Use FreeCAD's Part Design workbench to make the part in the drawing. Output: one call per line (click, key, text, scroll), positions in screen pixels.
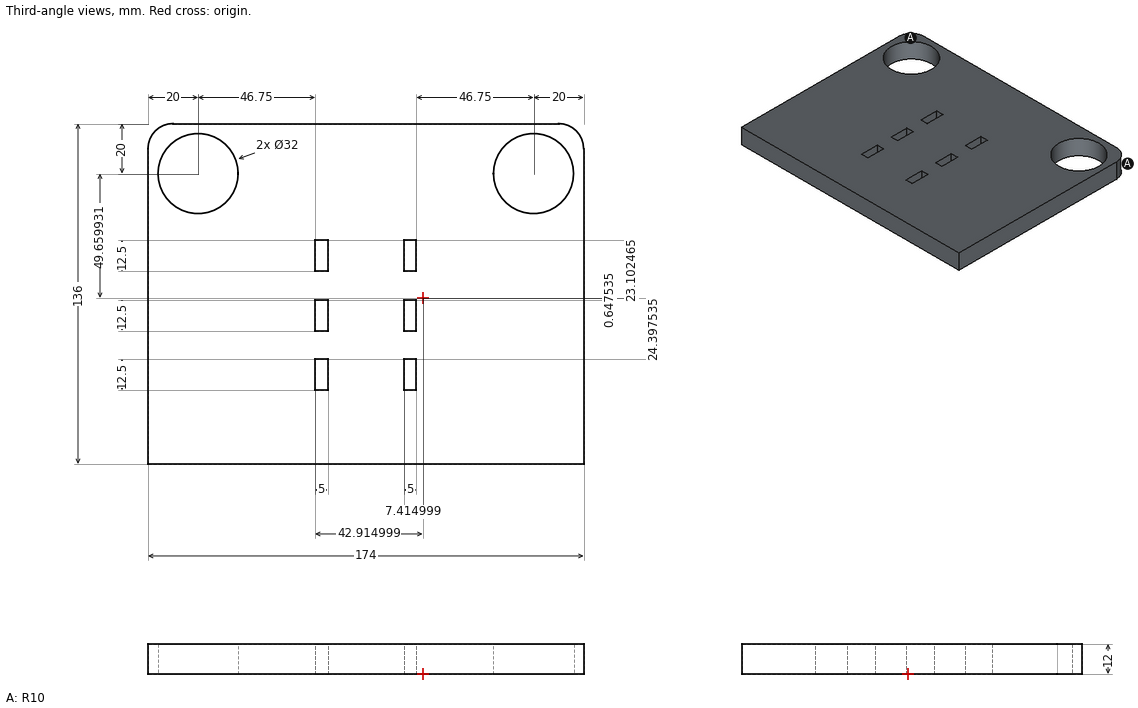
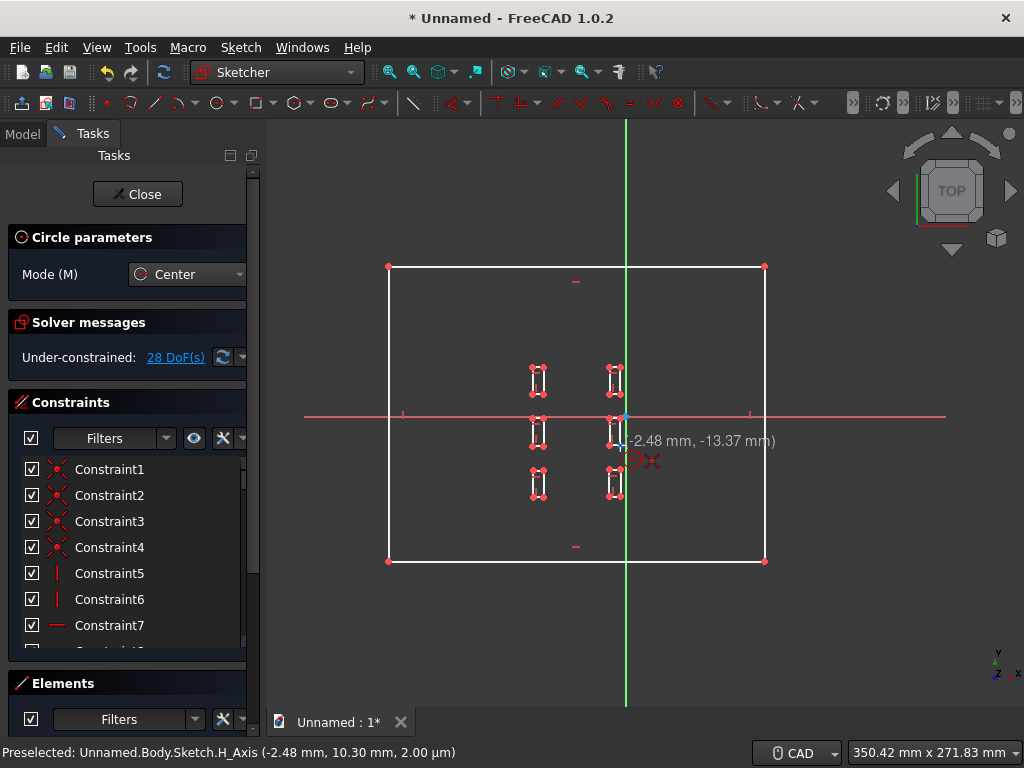
click(432, 309)
click(456, 285)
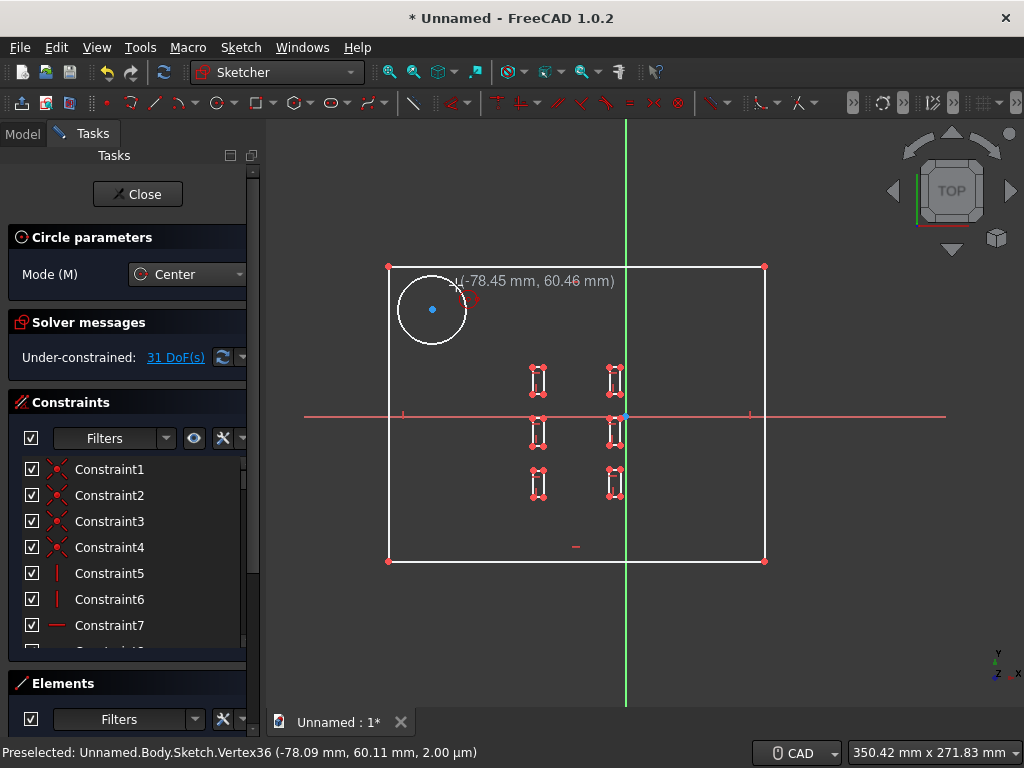
click(722, 309)
click(746, 285)
key(Escape)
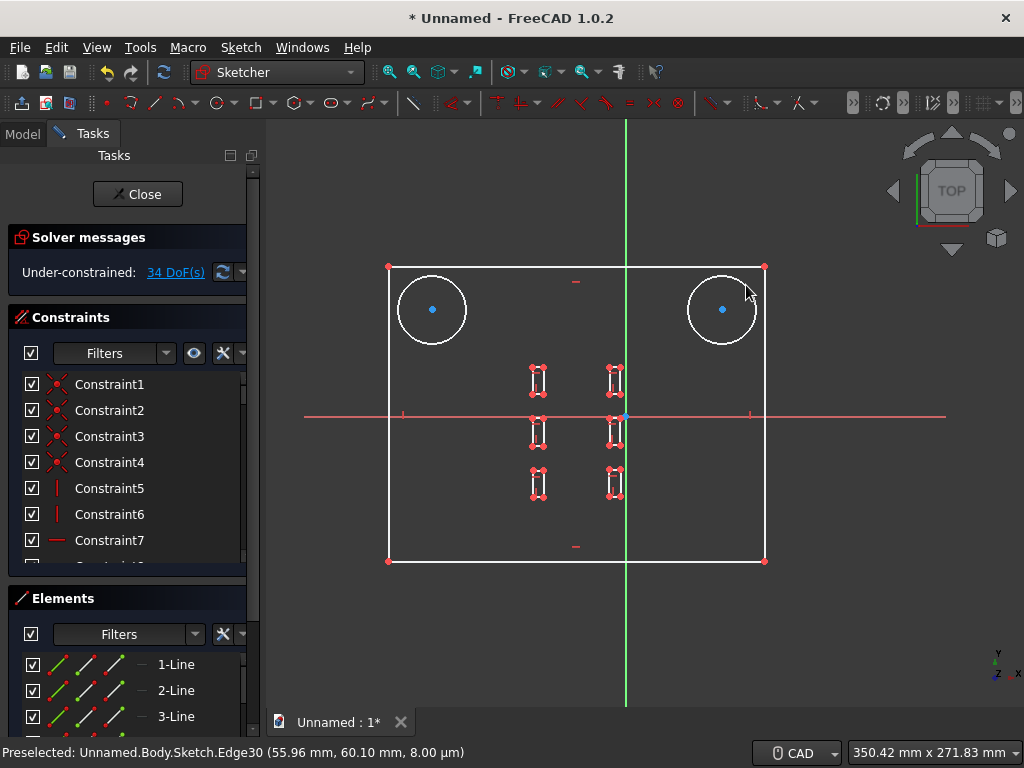
click(456, 286)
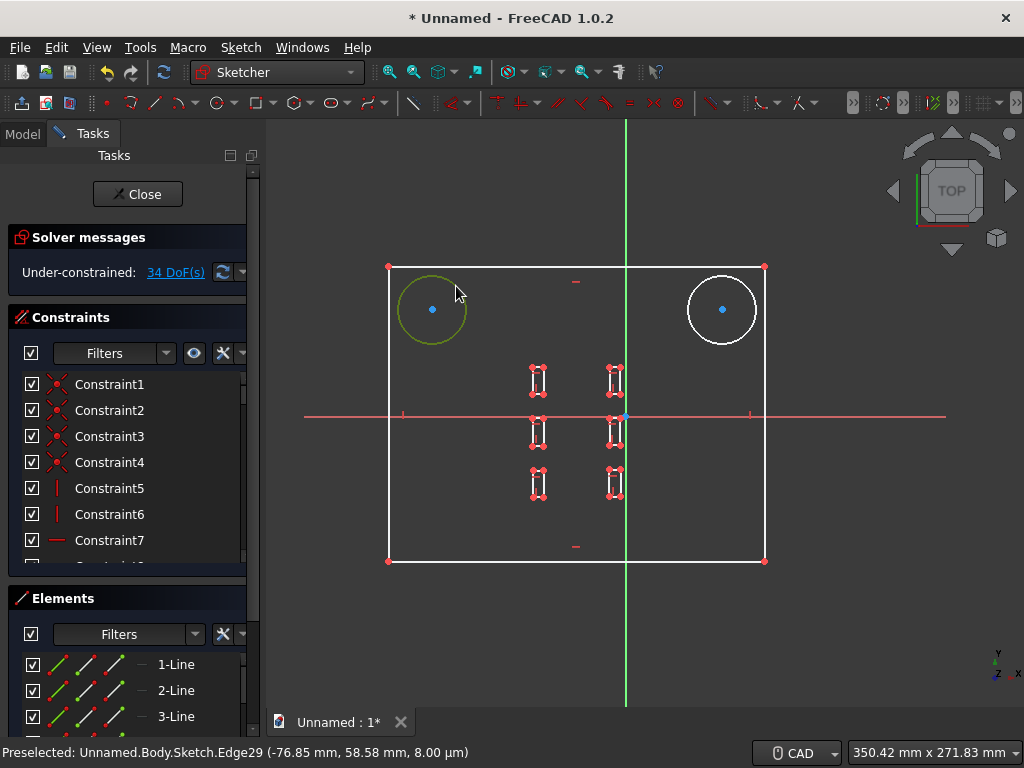
click(746, 286)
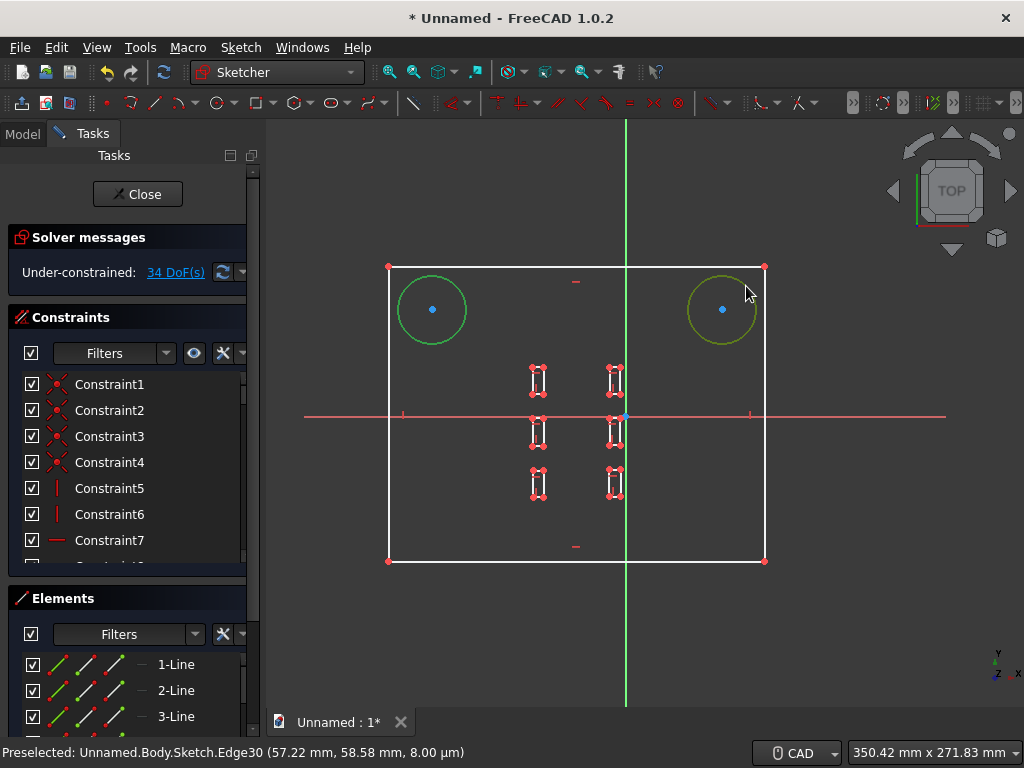
click(630, 104)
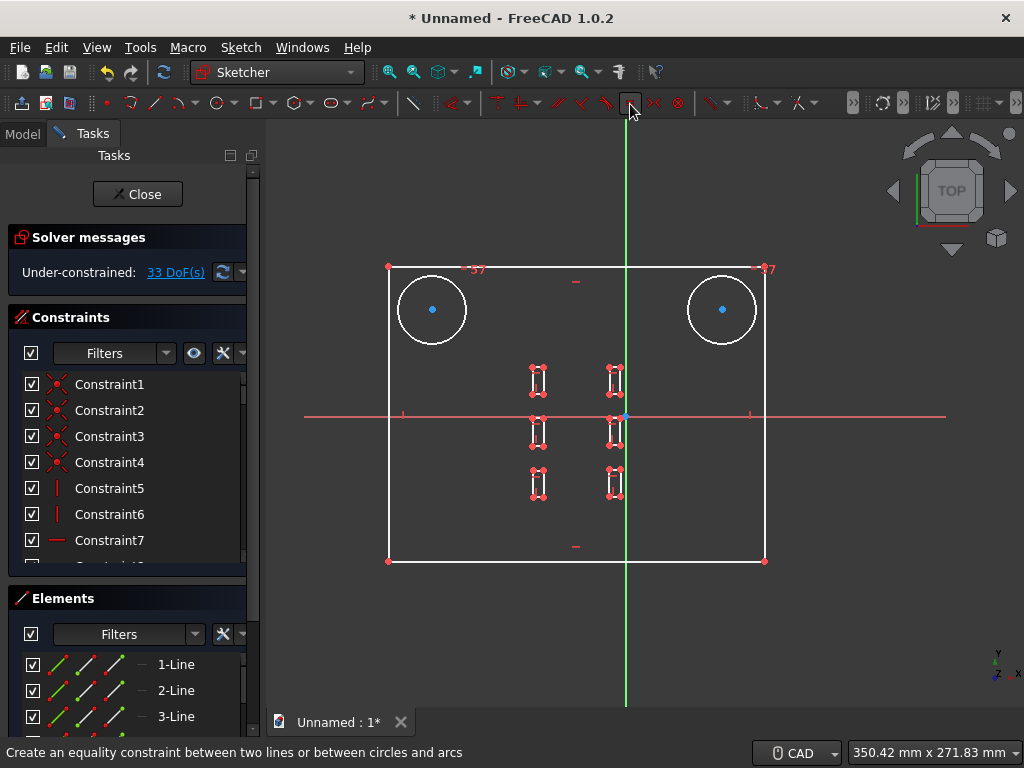
click(456, 286)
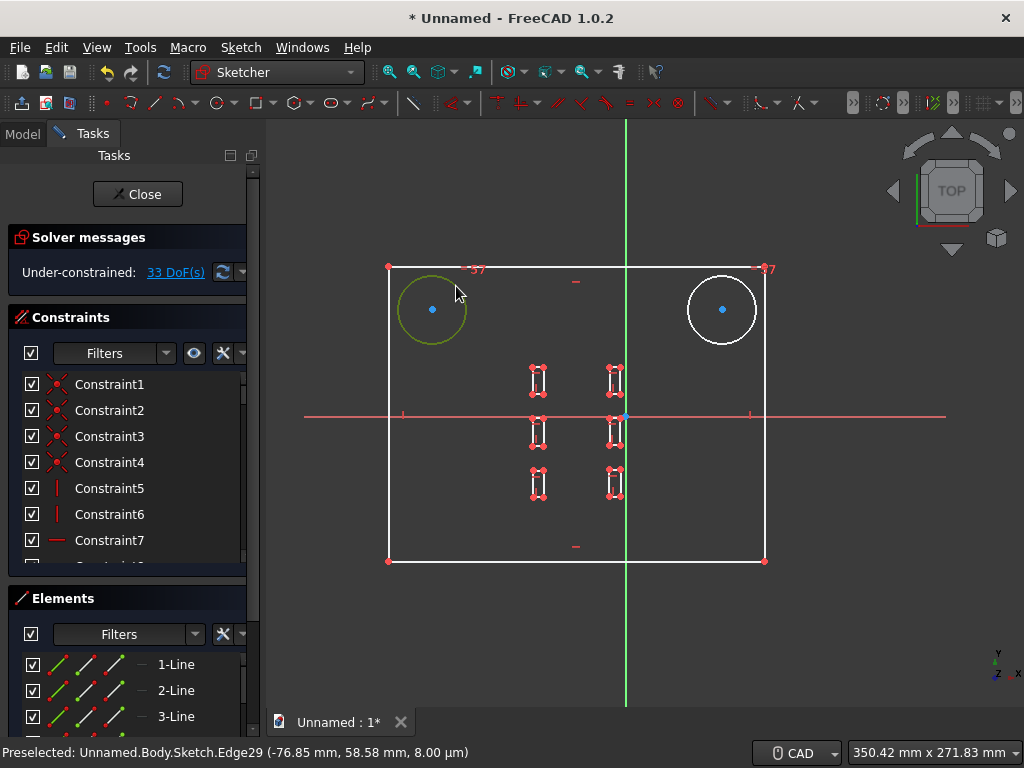
key(k)
key(o)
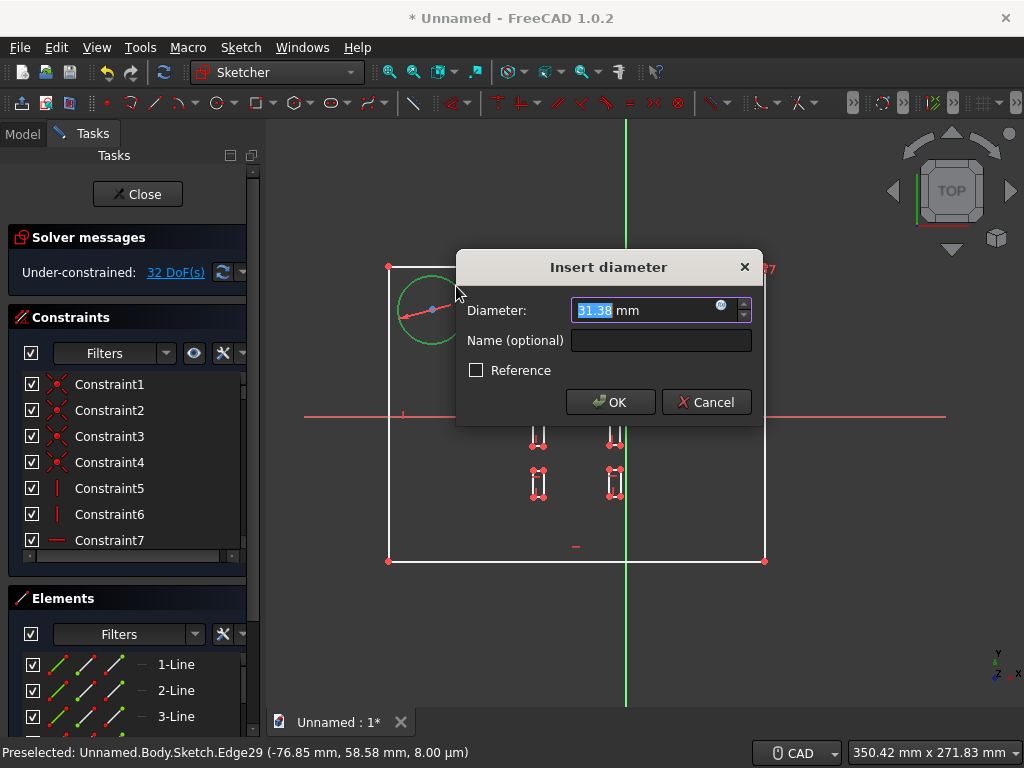
text(32)
key(Return)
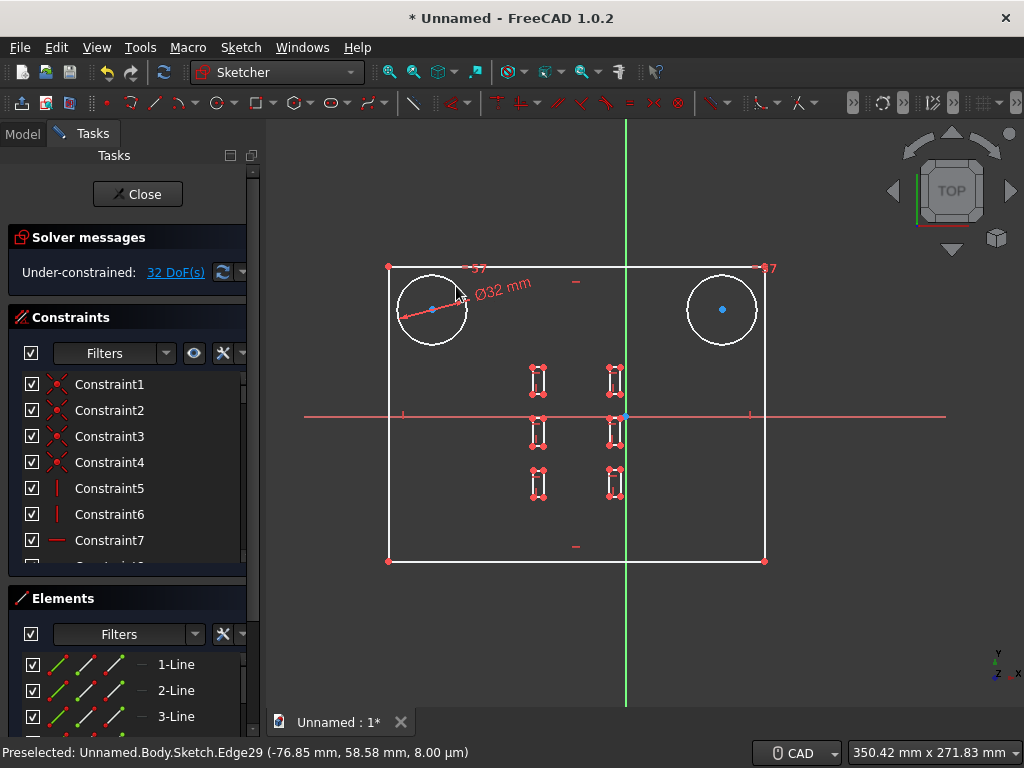
scroll(538, 497, up, 7)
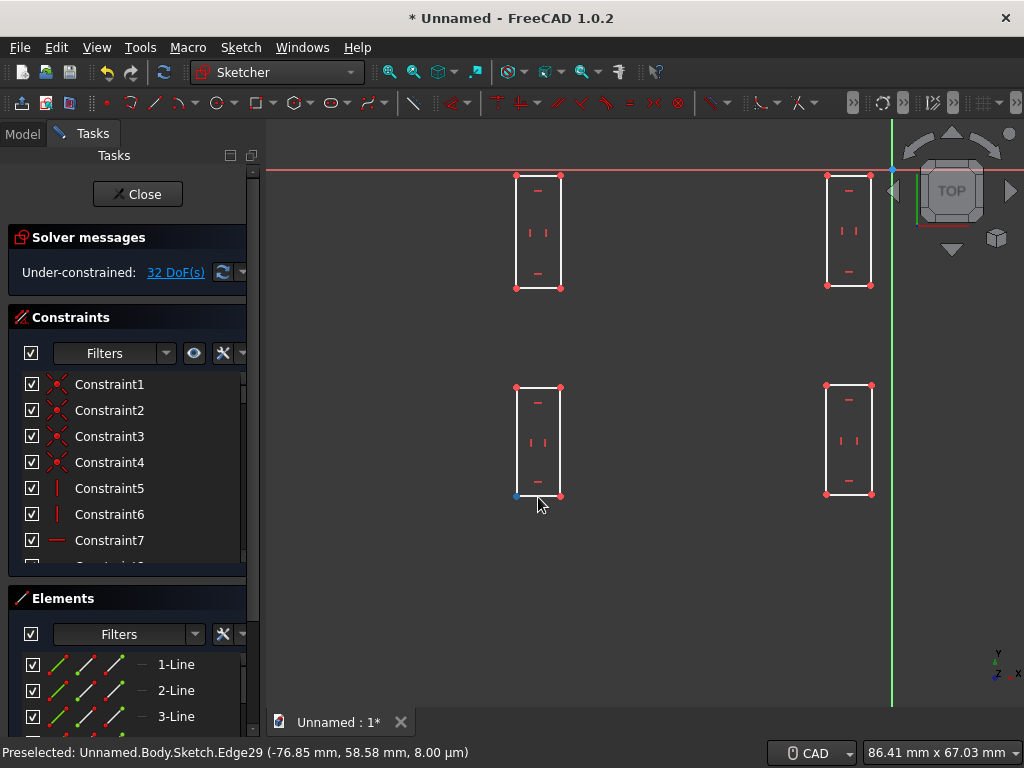
click(539, 496)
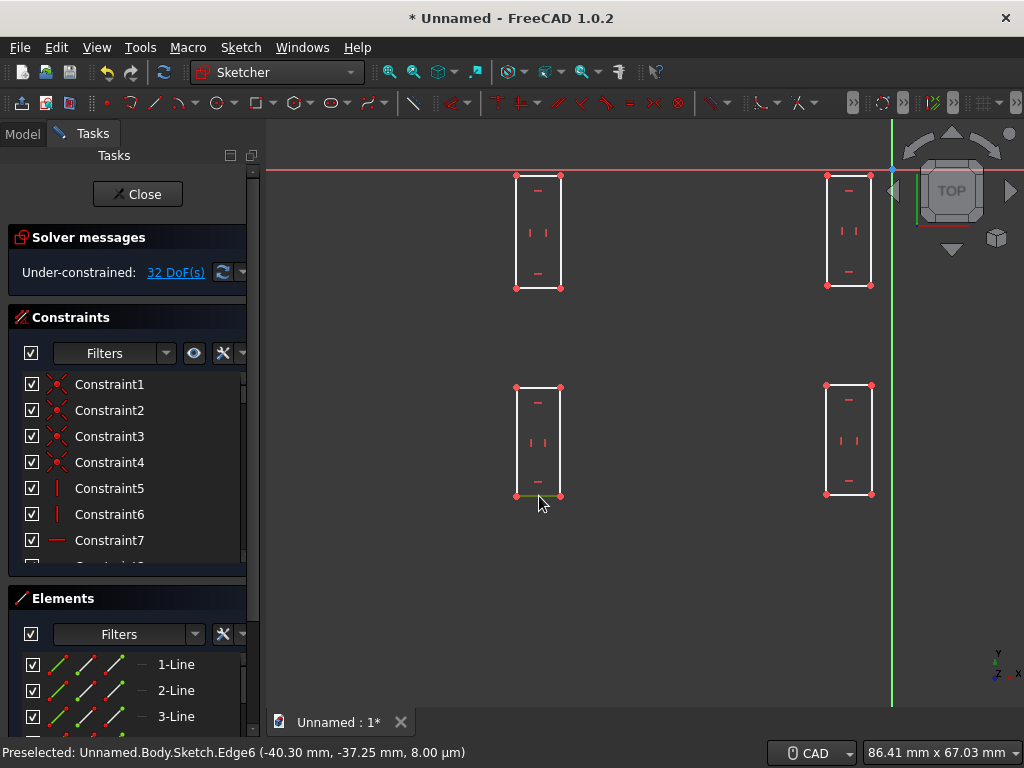
click(470, 104)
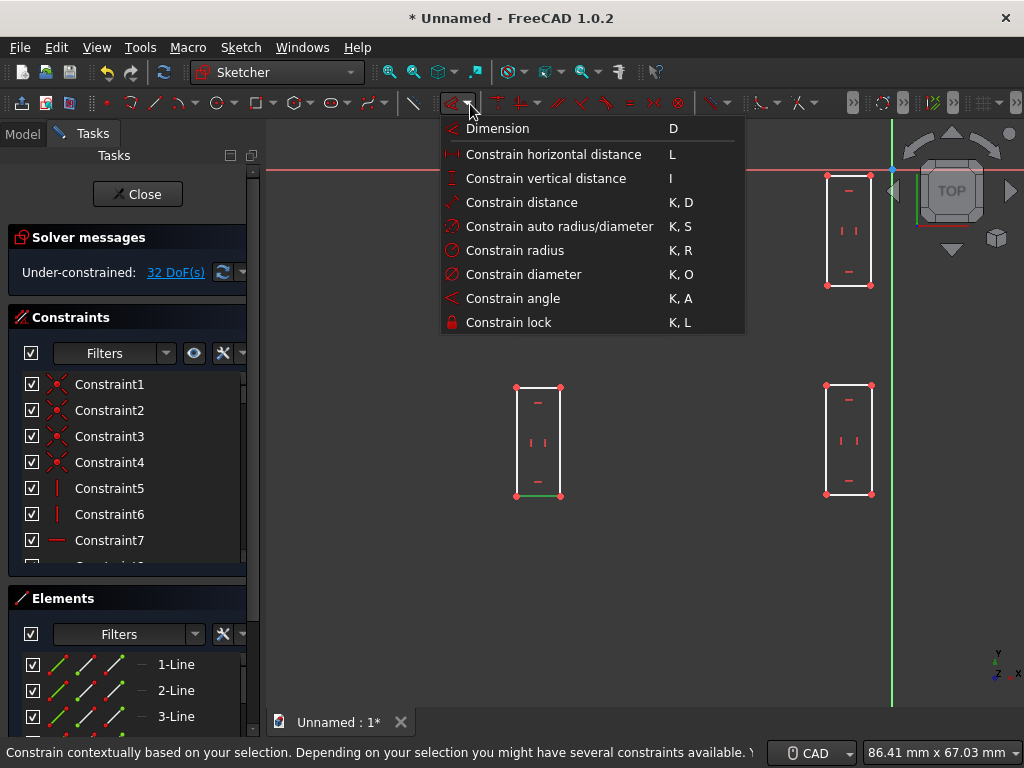
click(593, 154)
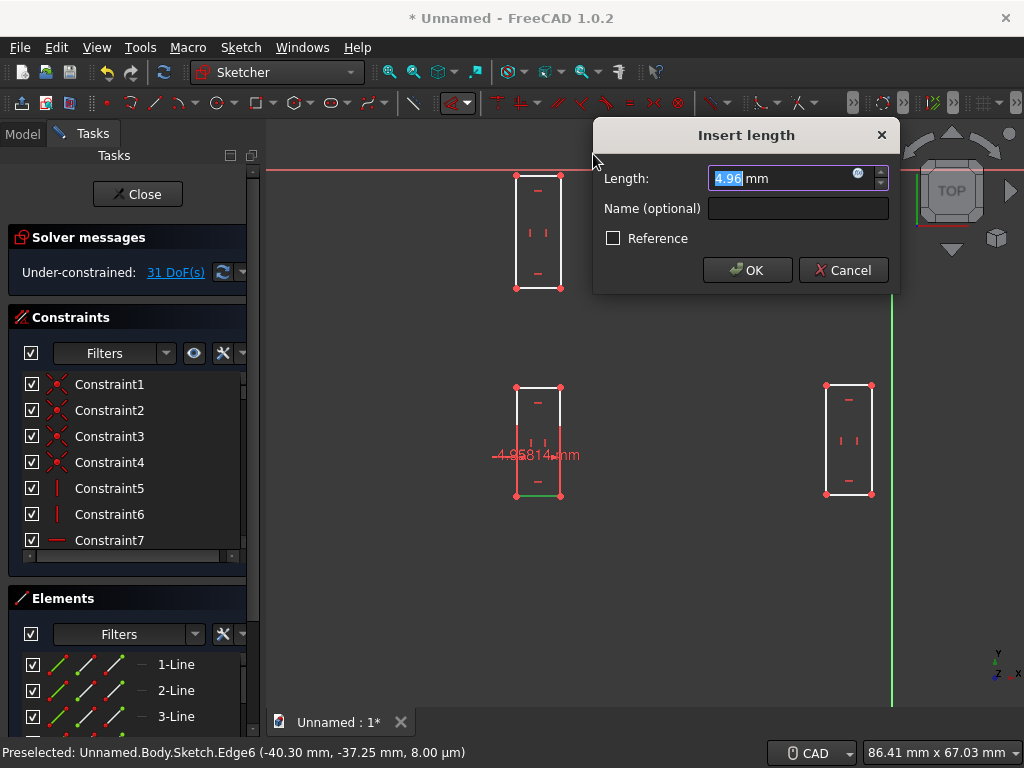
text(5)
key(Return)